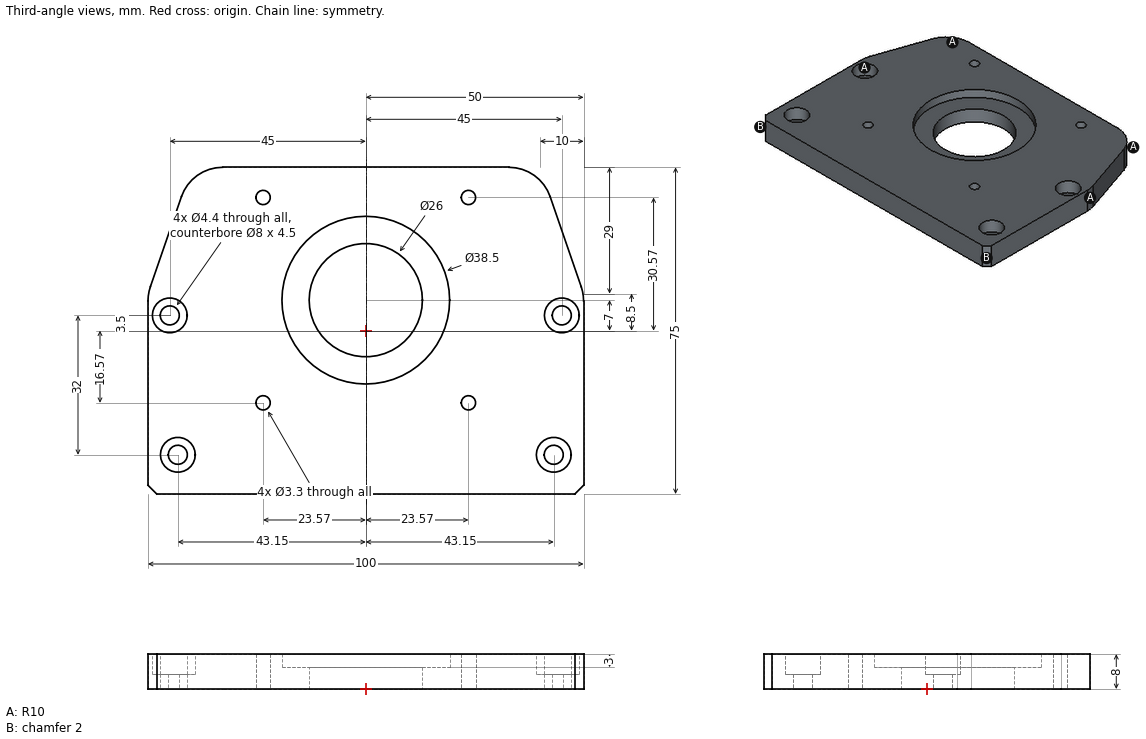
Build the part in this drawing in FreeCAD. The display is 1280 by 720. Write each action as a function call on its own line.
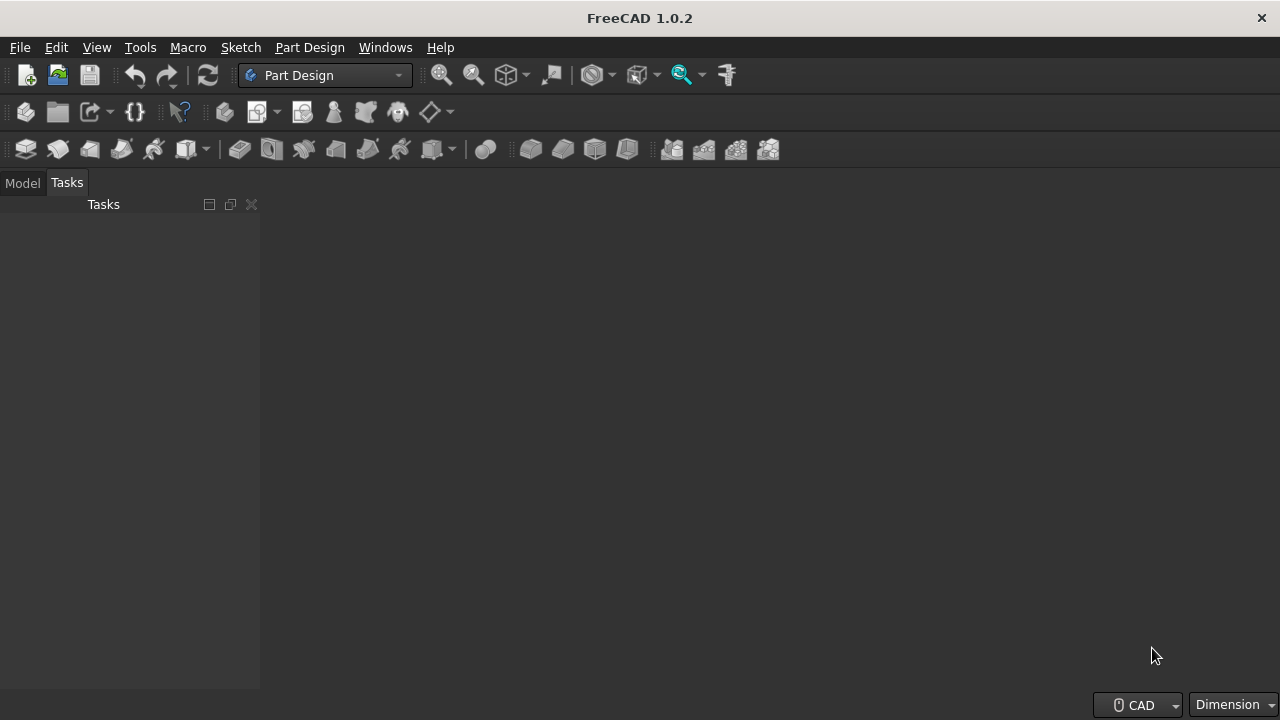
click(26, 76)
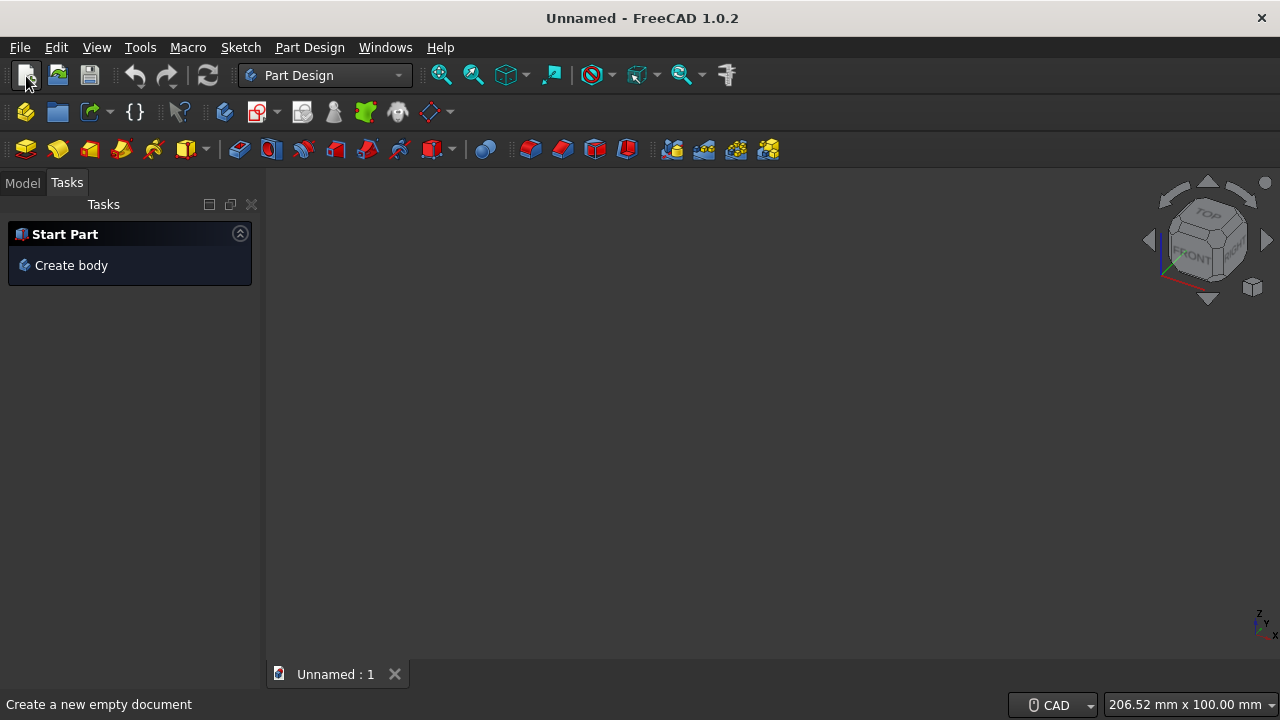
click(258, 112)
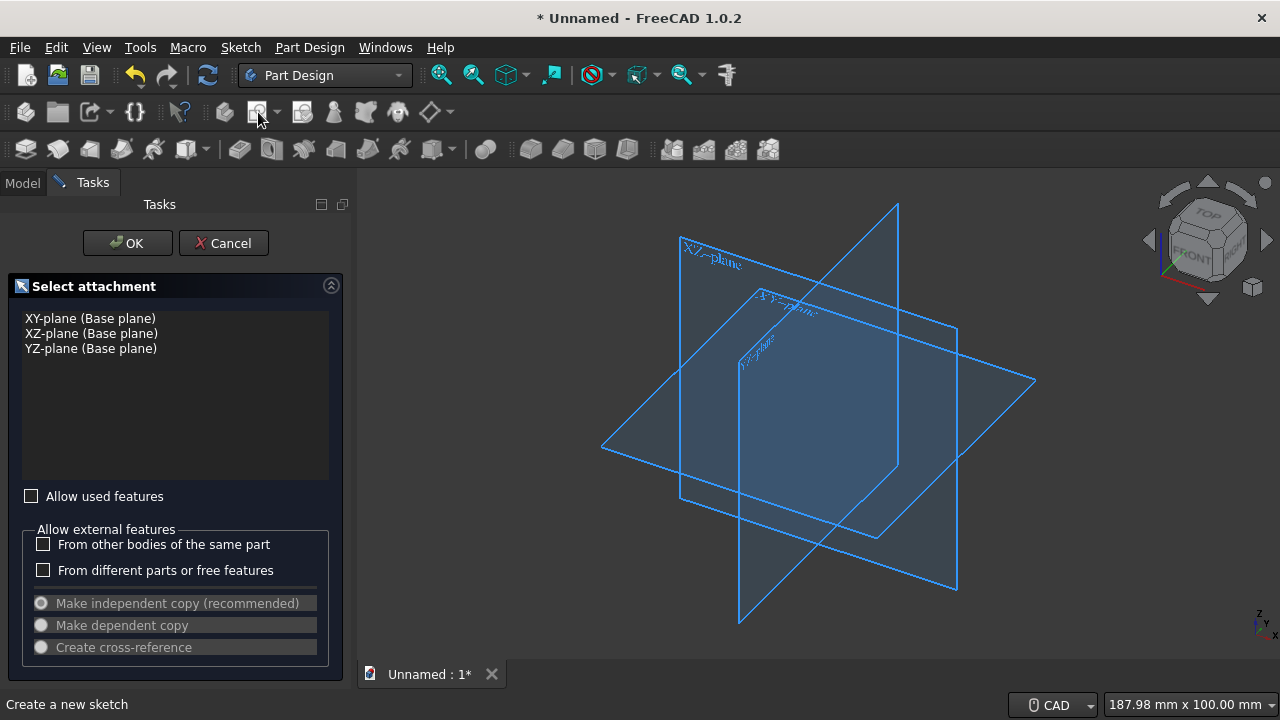
click(82, 318)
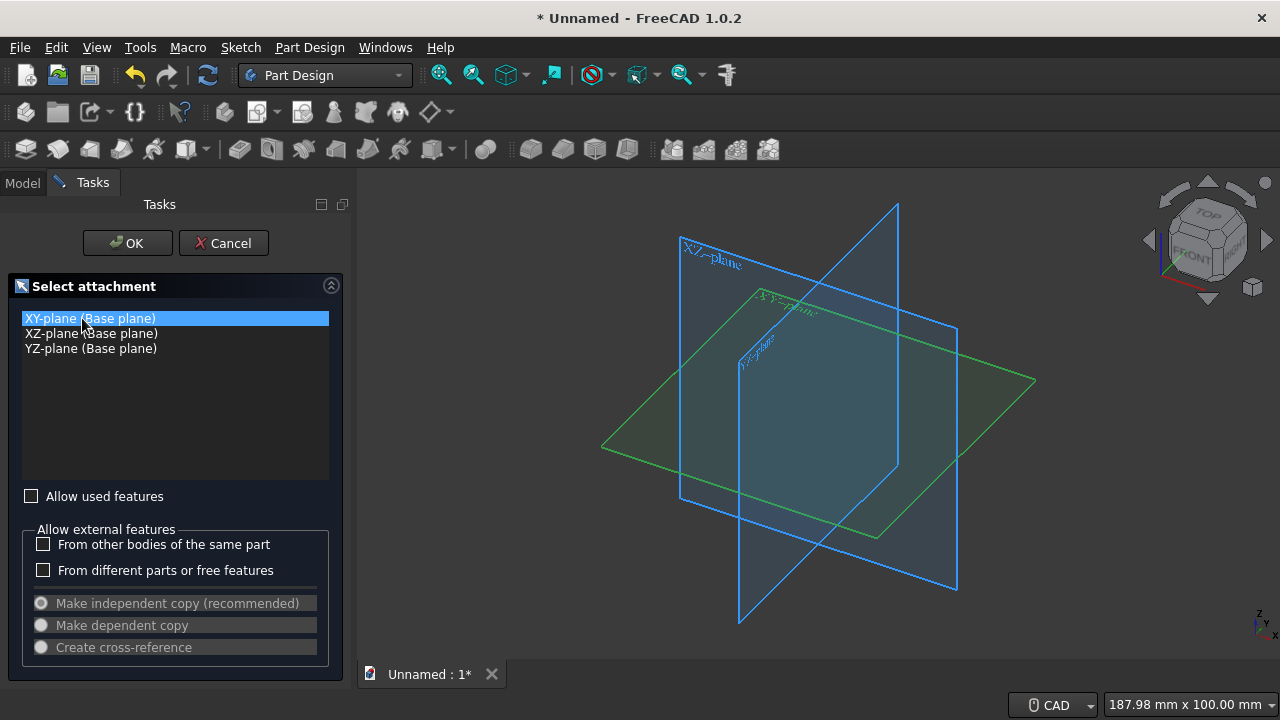
click(128, 243)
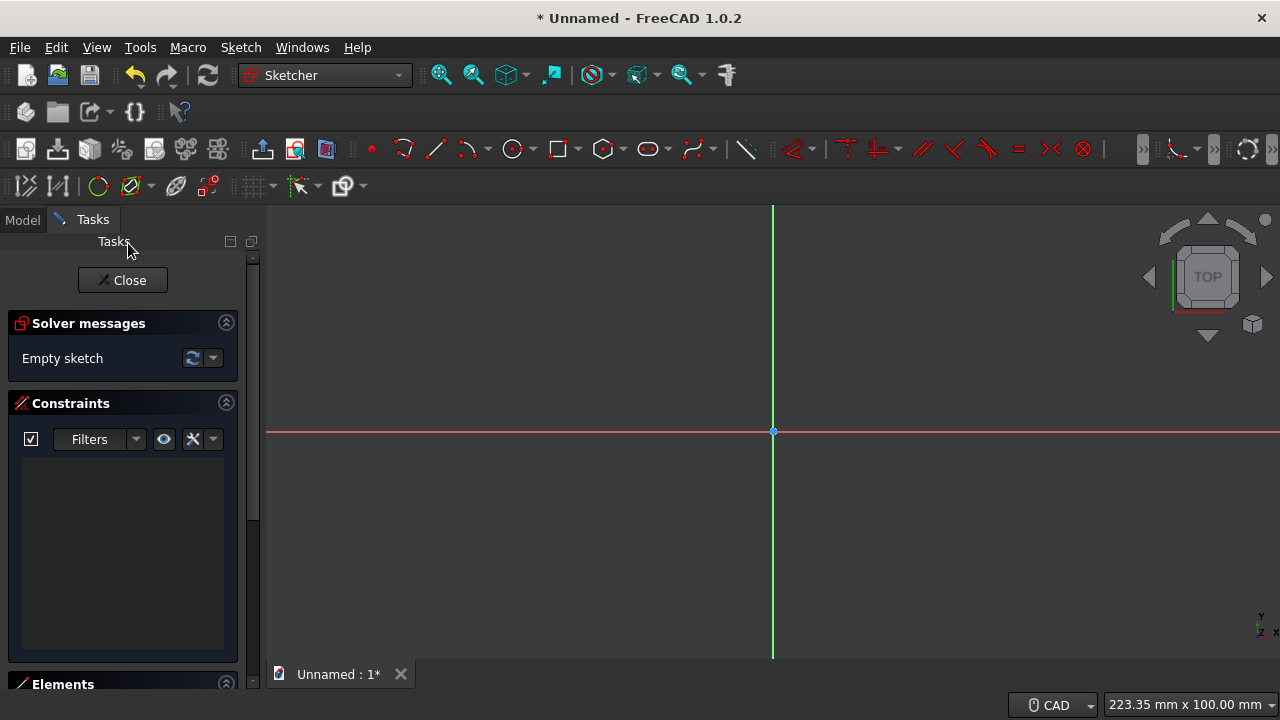
click(580, 150)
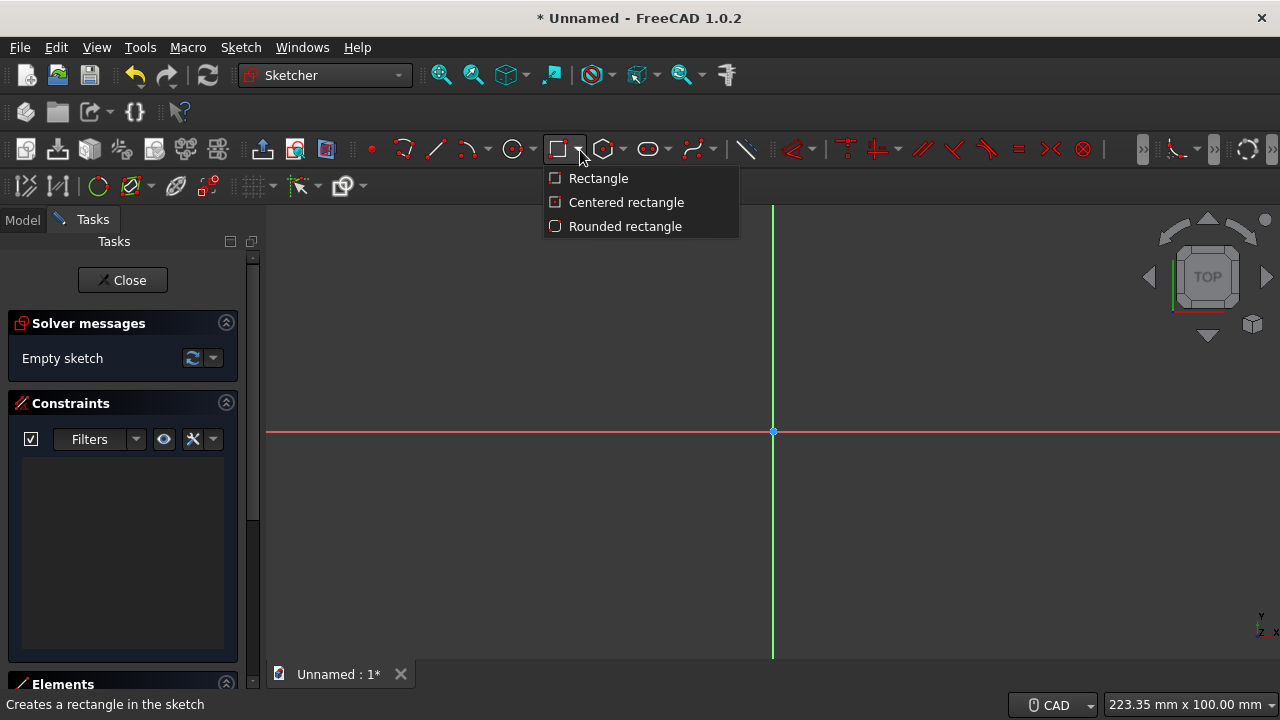
click(642, 202)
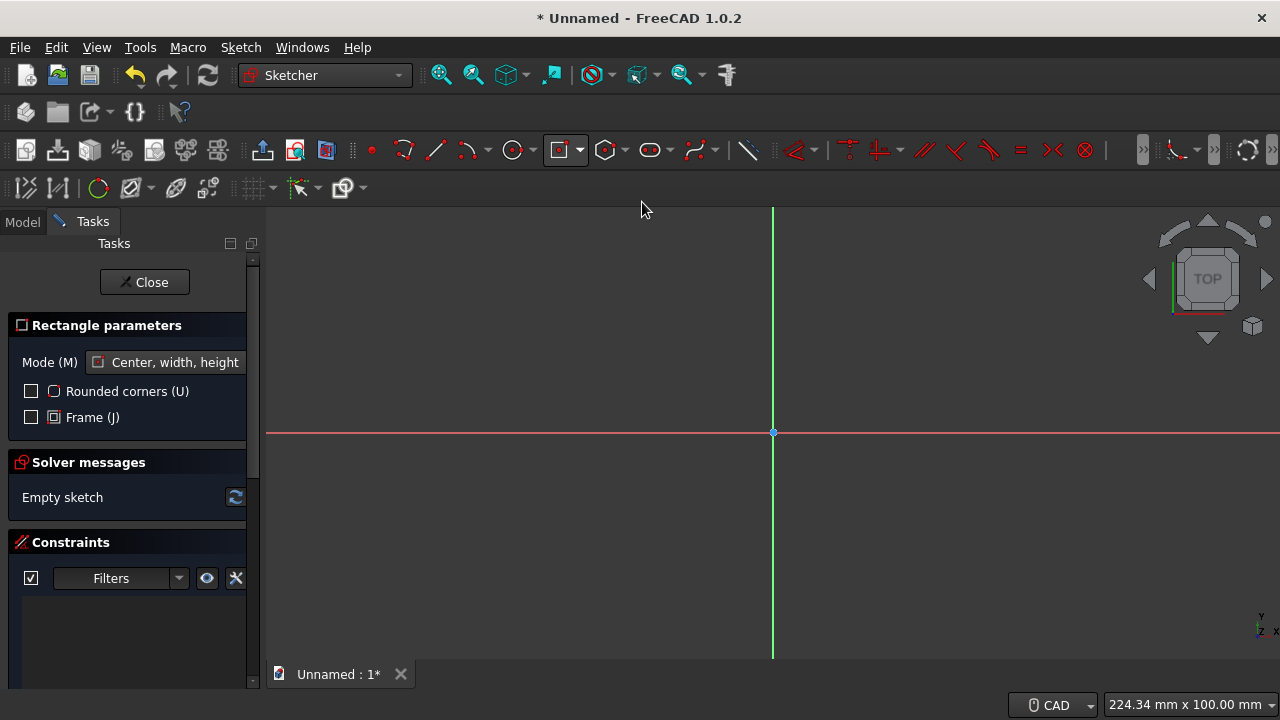
click(773, 433)
click(999, 264)
key(Escape)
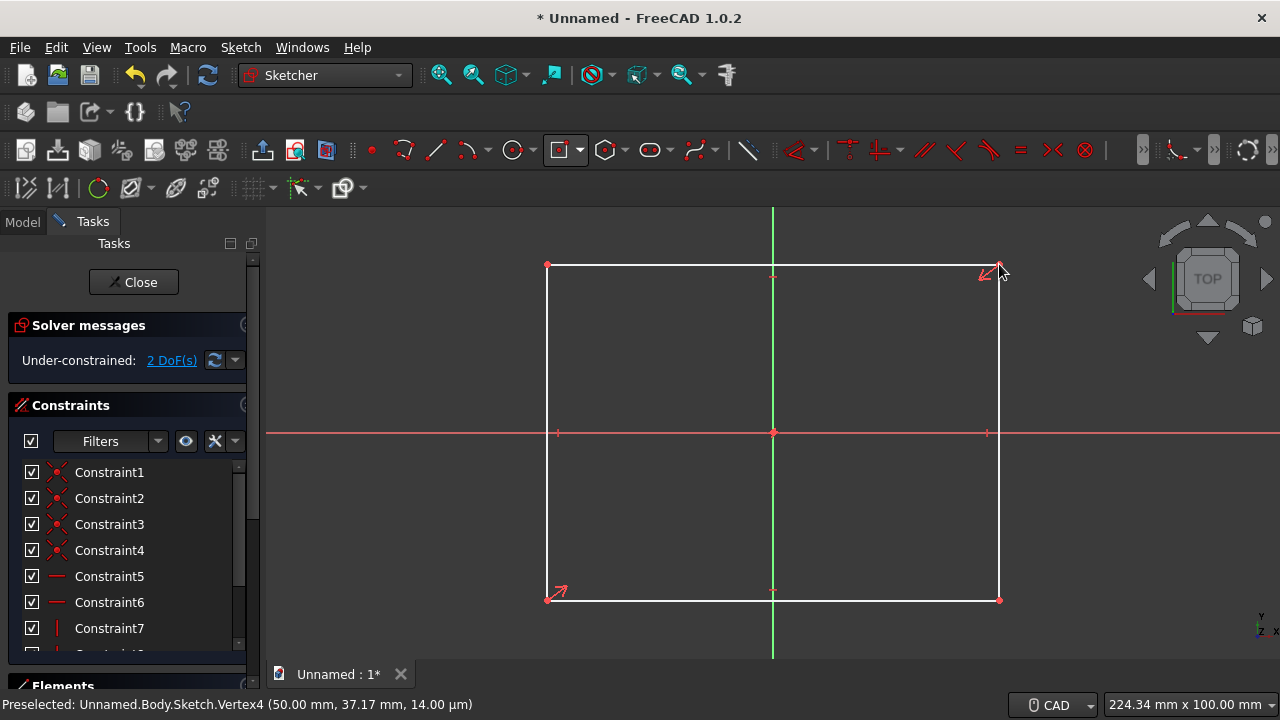
click(999, 500)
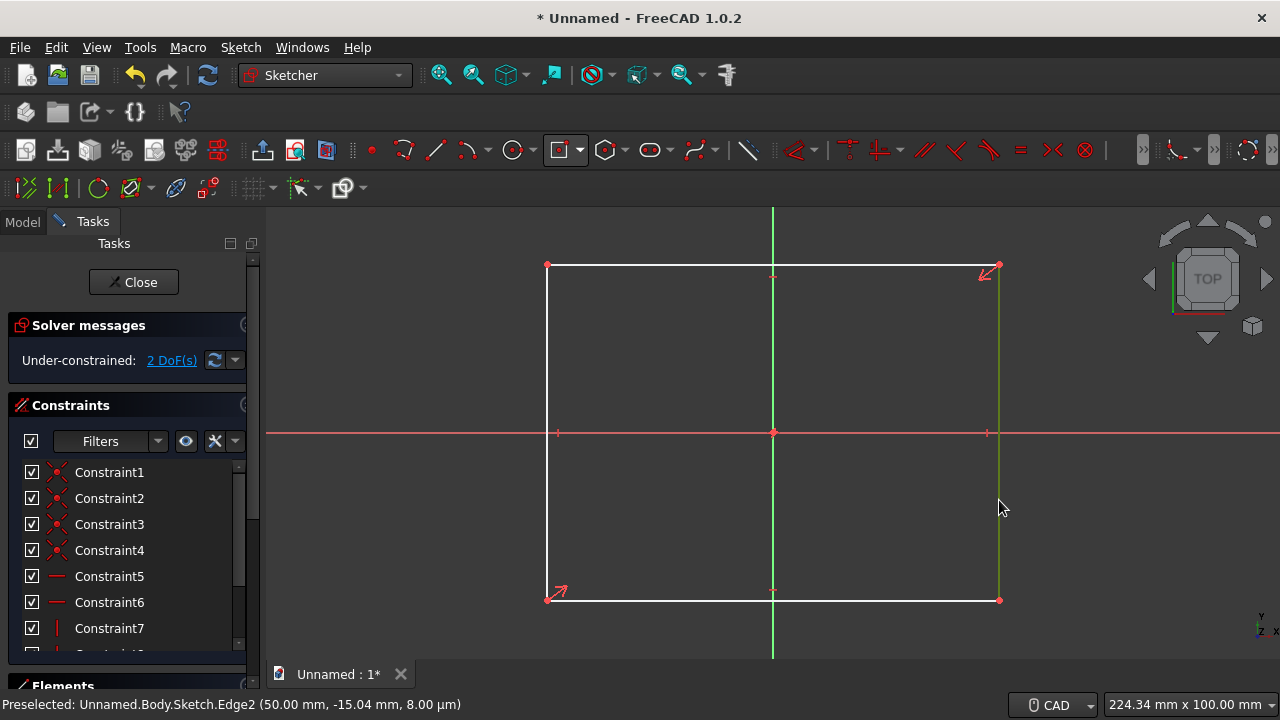
key(i)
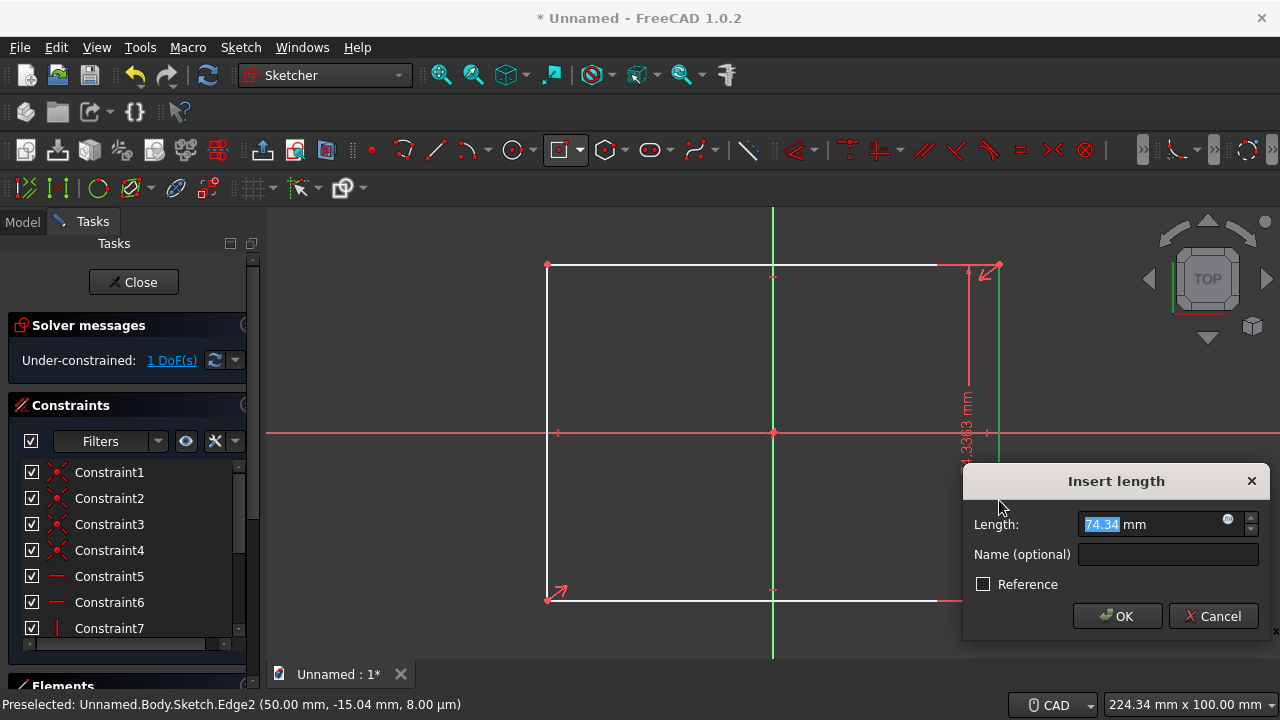
text(75)
key(Return)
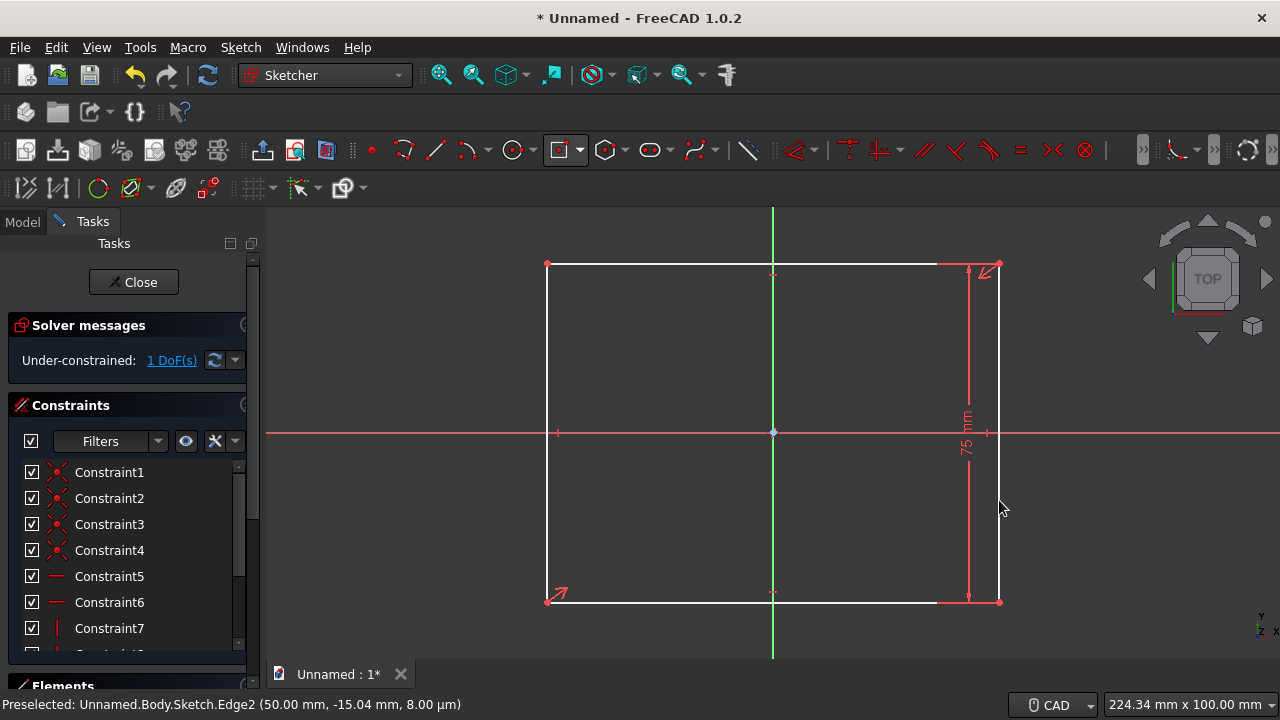
click(683, 602)